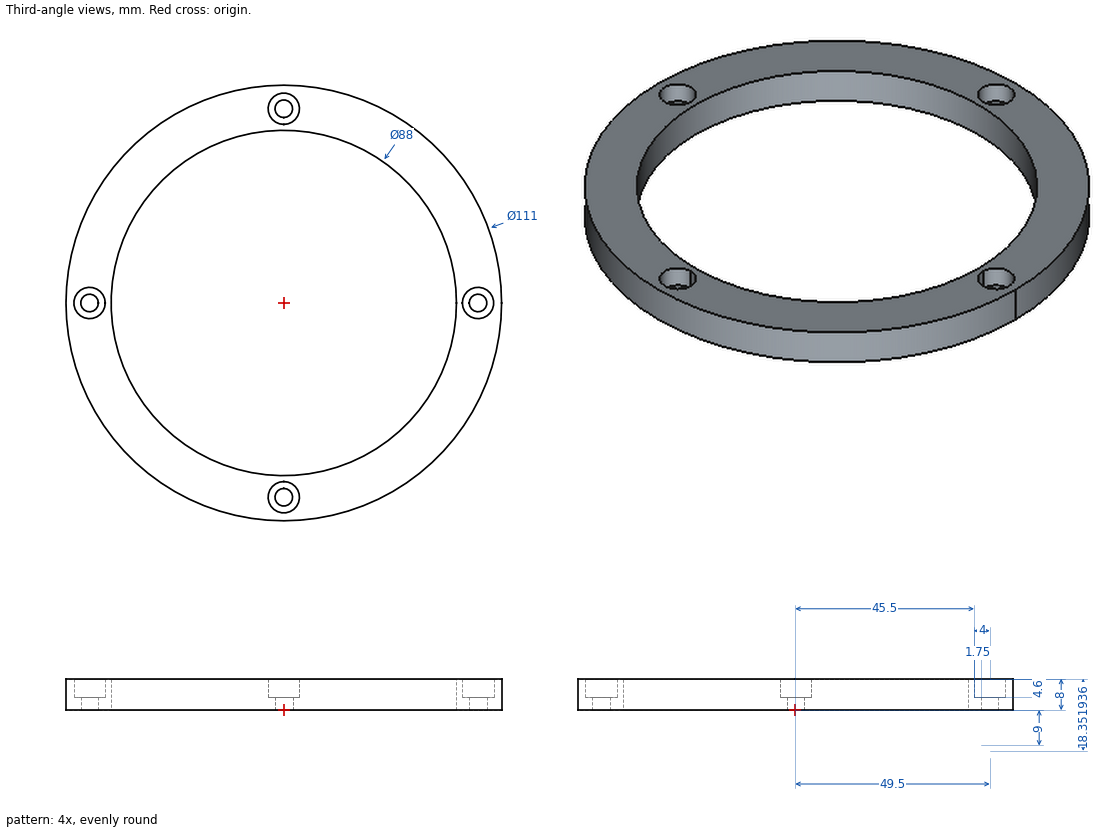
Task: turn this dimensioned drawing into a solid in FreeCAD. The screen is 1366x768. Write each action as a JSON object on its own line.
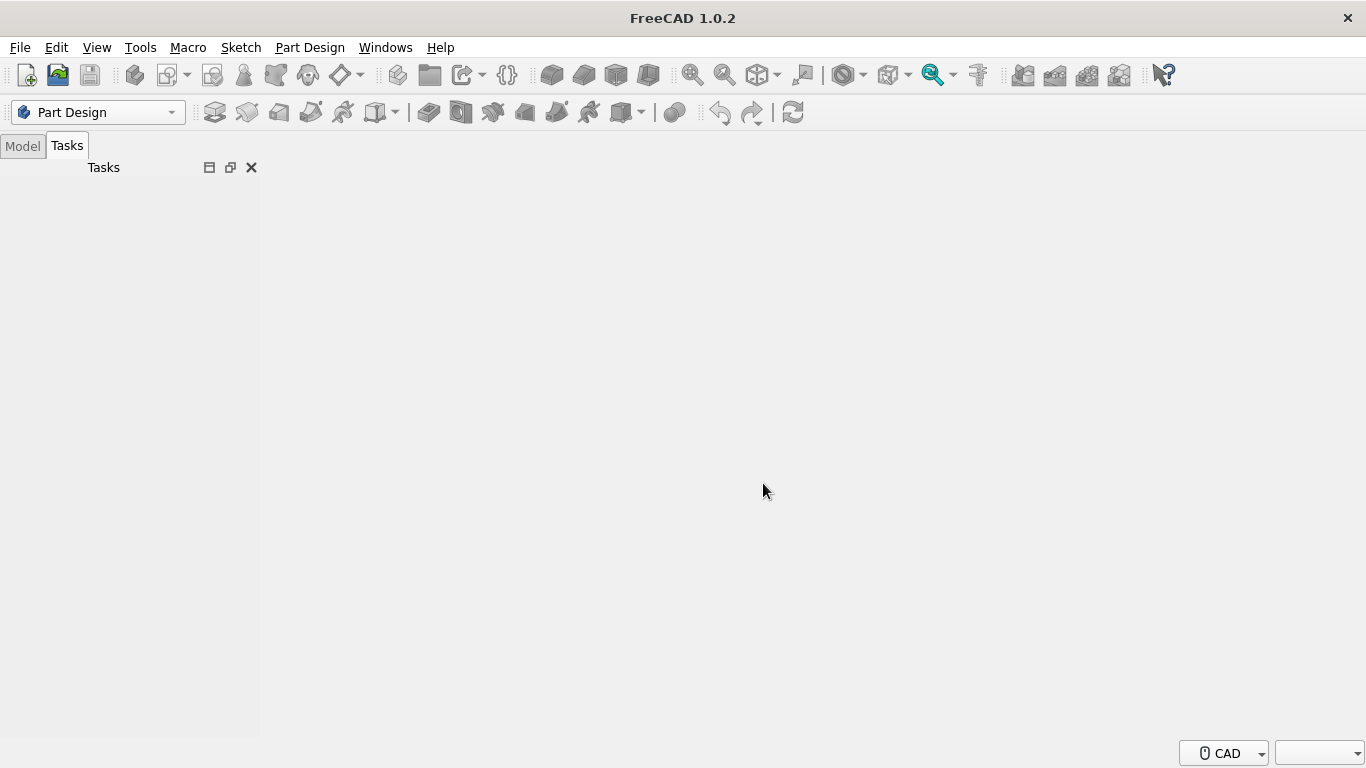
{"action": "left_click", "coordinate": [26, 76]}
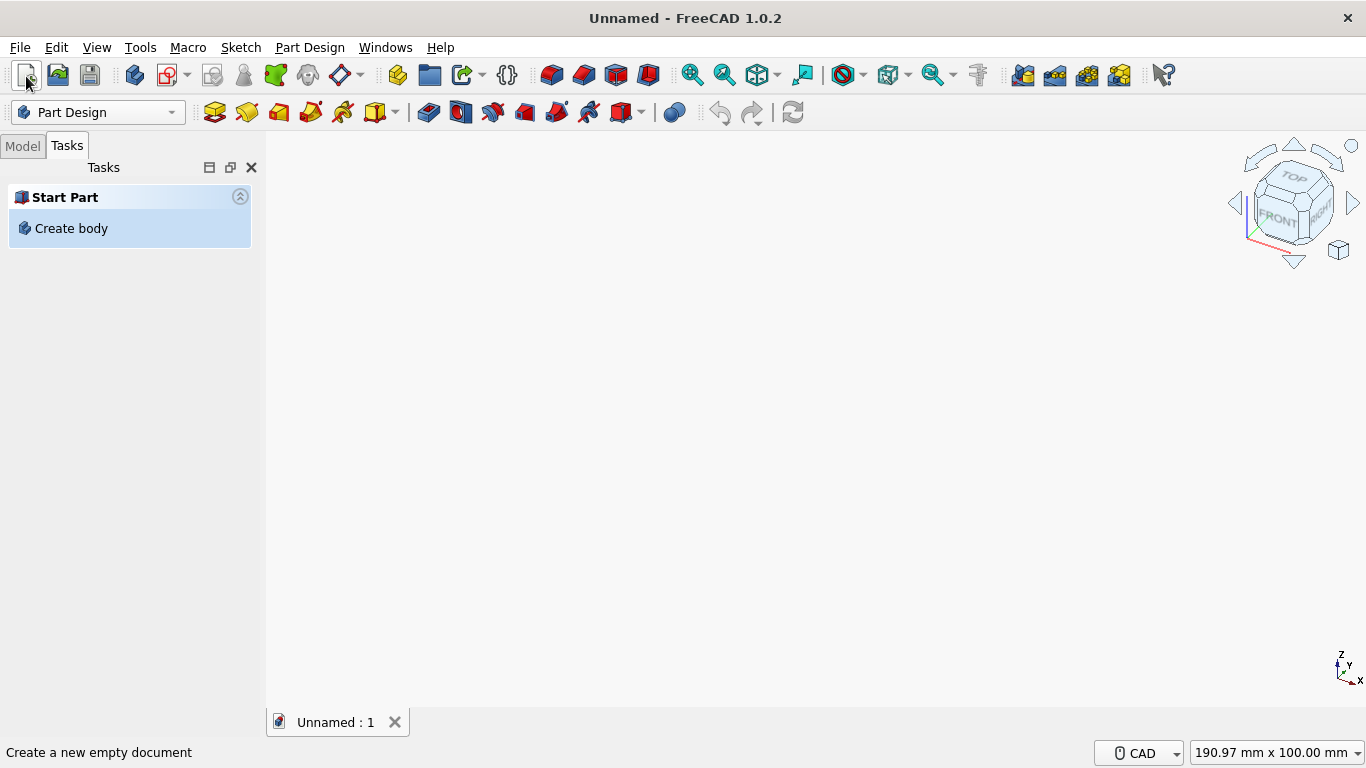
{"action": "left_click", "coordinate": [168, 76]}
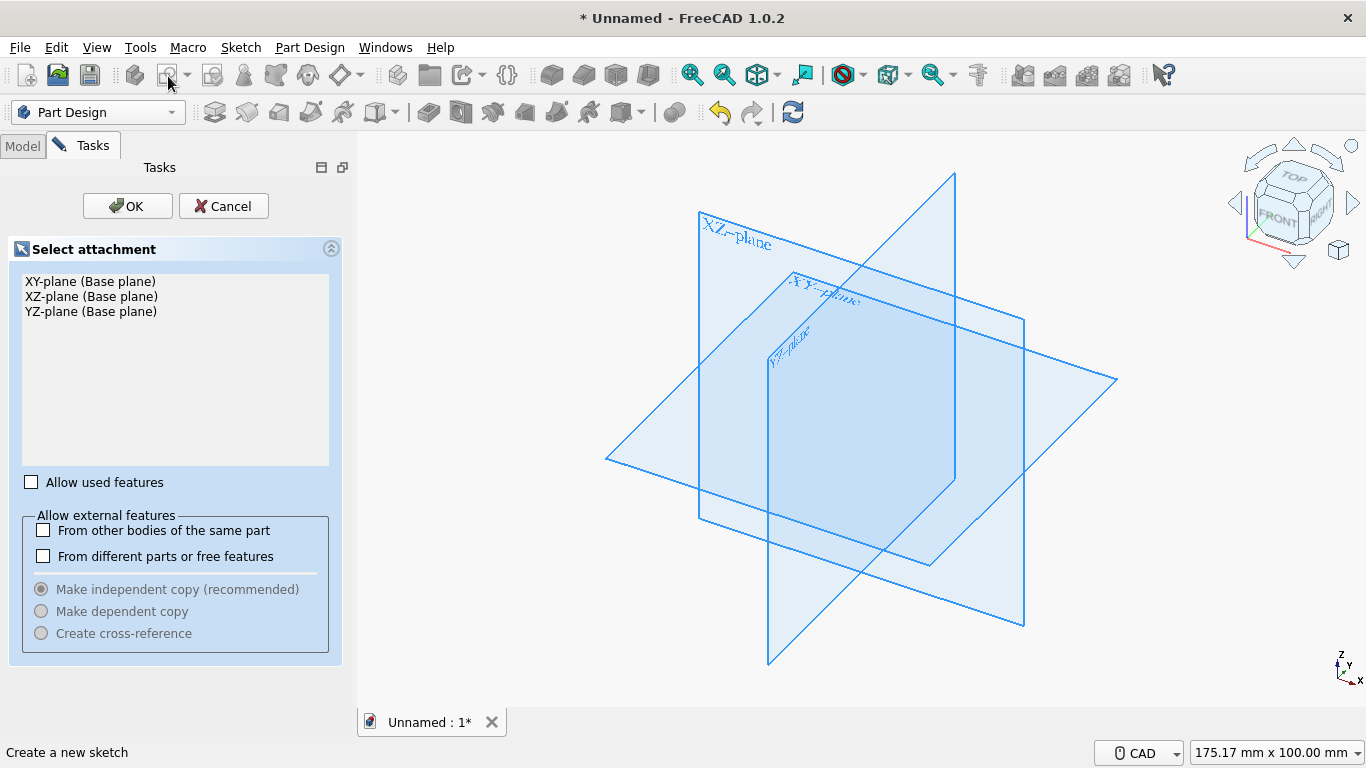
{"action": "left_click", "coordinate": [82, 282]}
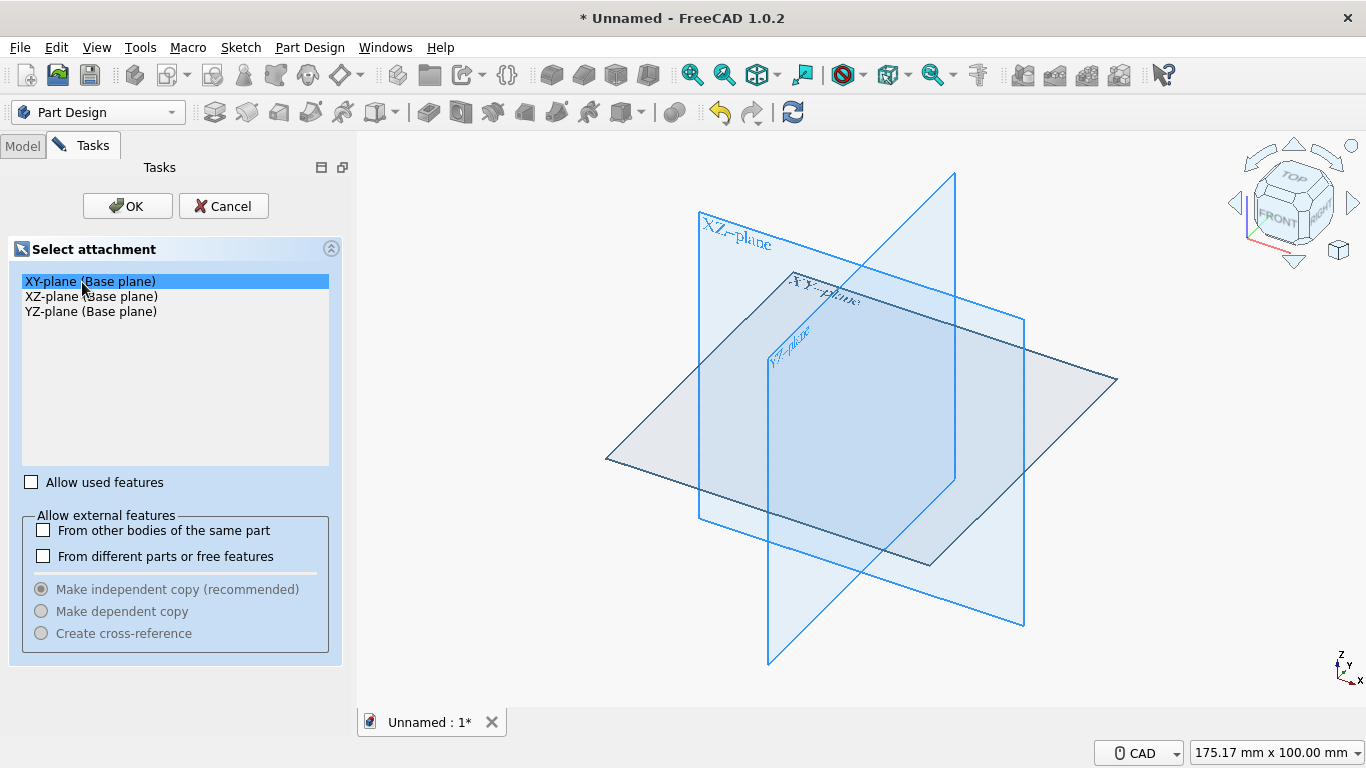
{"action": "left_click", "coordinate": [128, 206]}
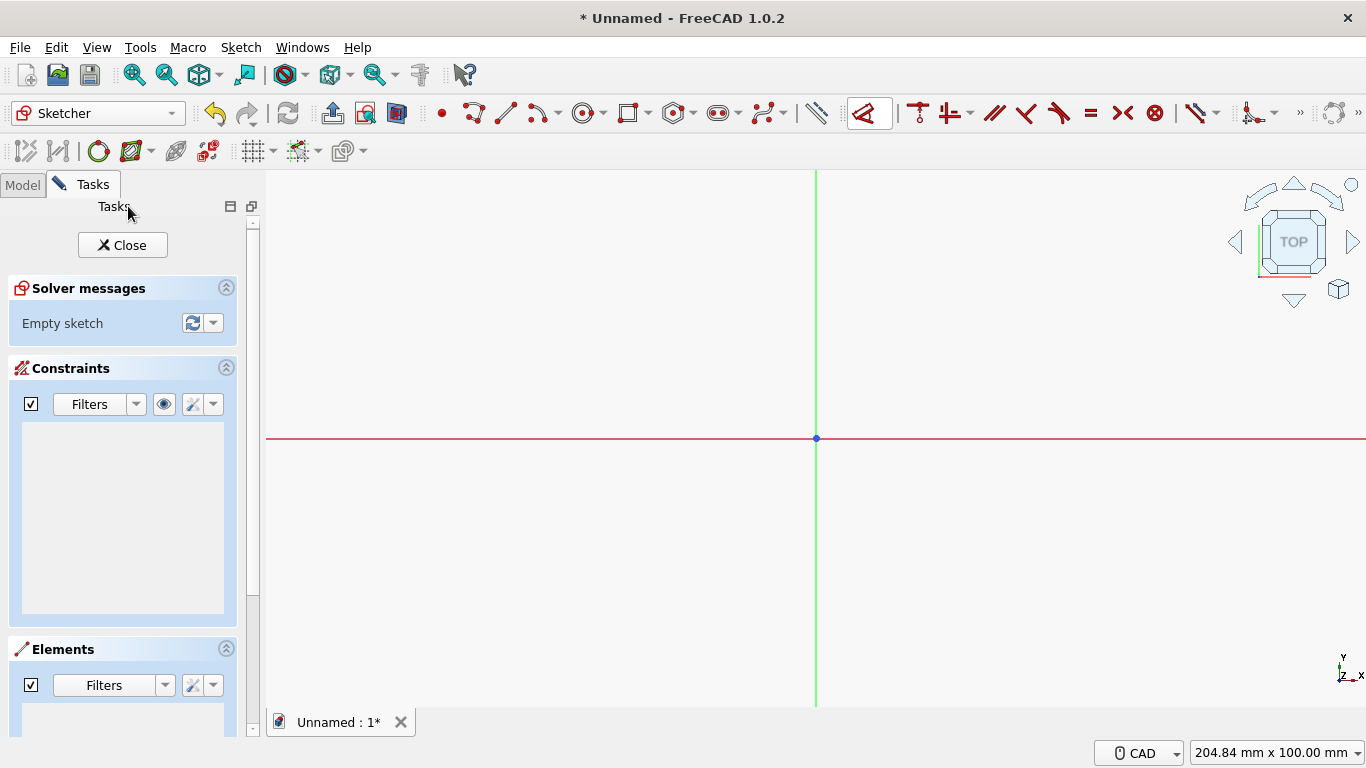
{"action": "scroll", "coordinate": [664, 438], "scroll_direction": "down", "scroll_amount": 3}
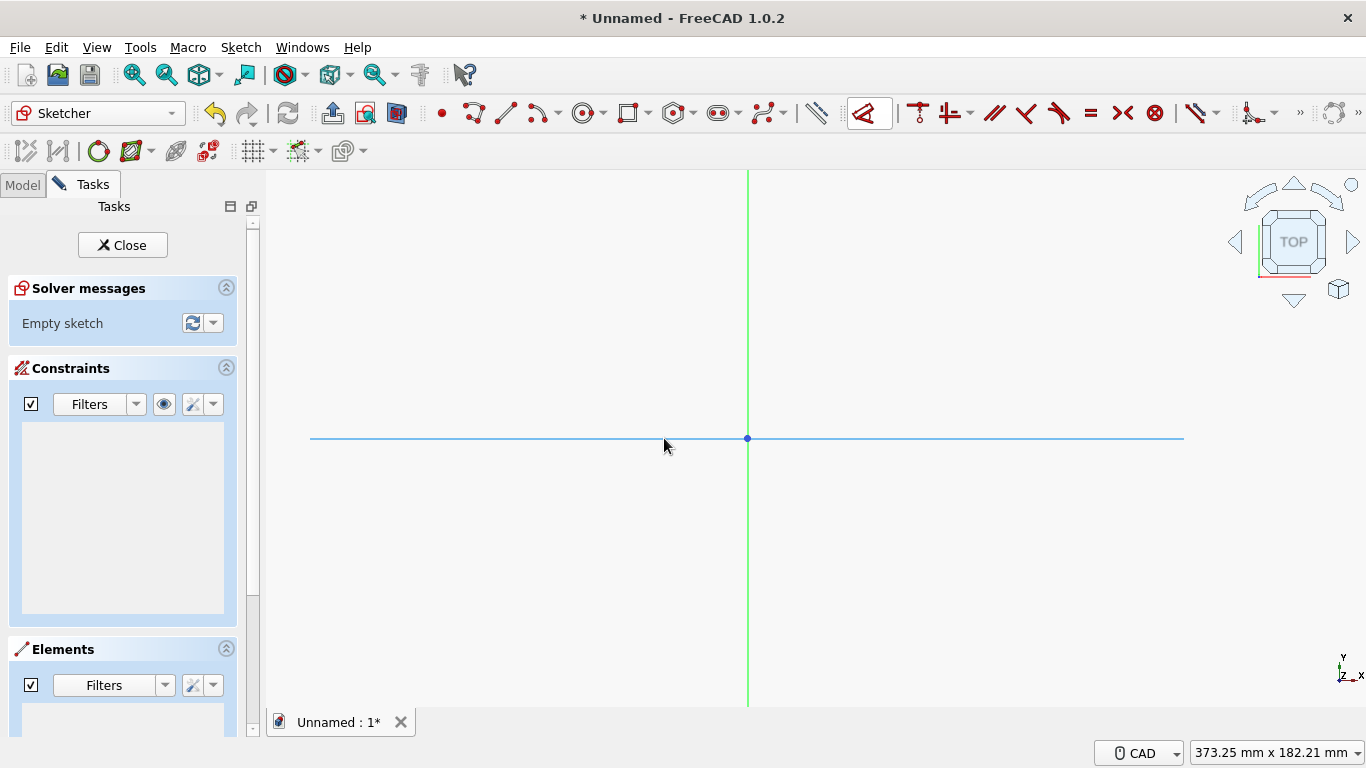
{"action": "key", "text": "g c"}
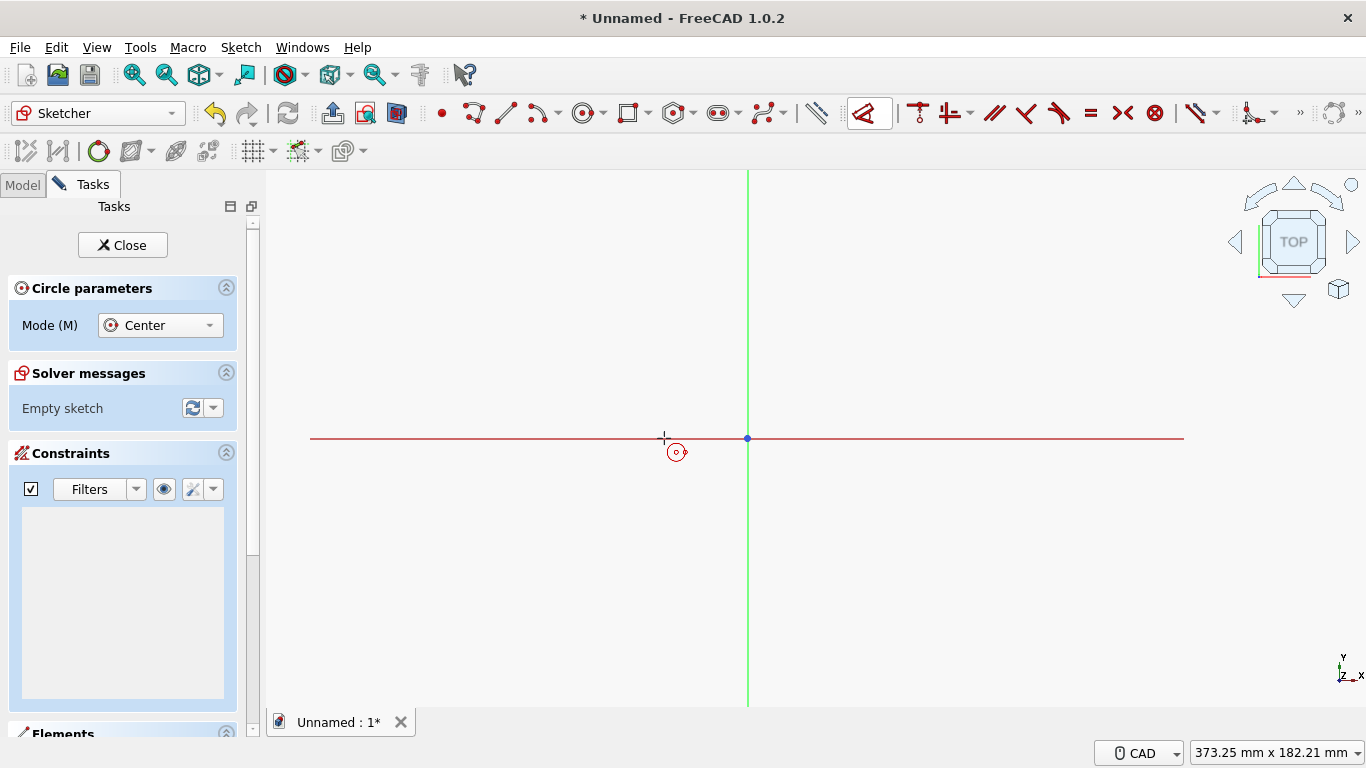
{"action": "left_click", "coordinate": [748, 438]}
{"action": "mouse_move", "coordinate": [863, 323]}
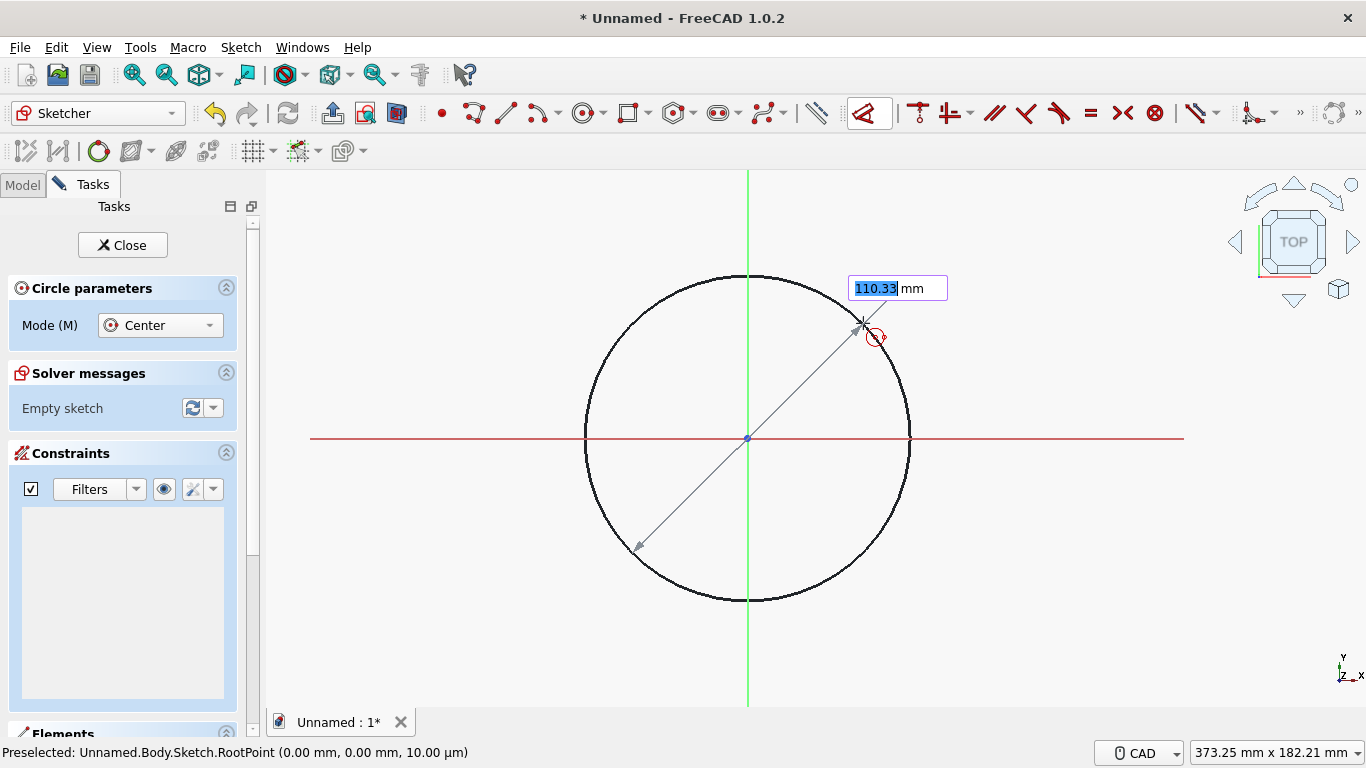
{"action": "type", "text": "111"}
{"action": "key", "text": "Return"}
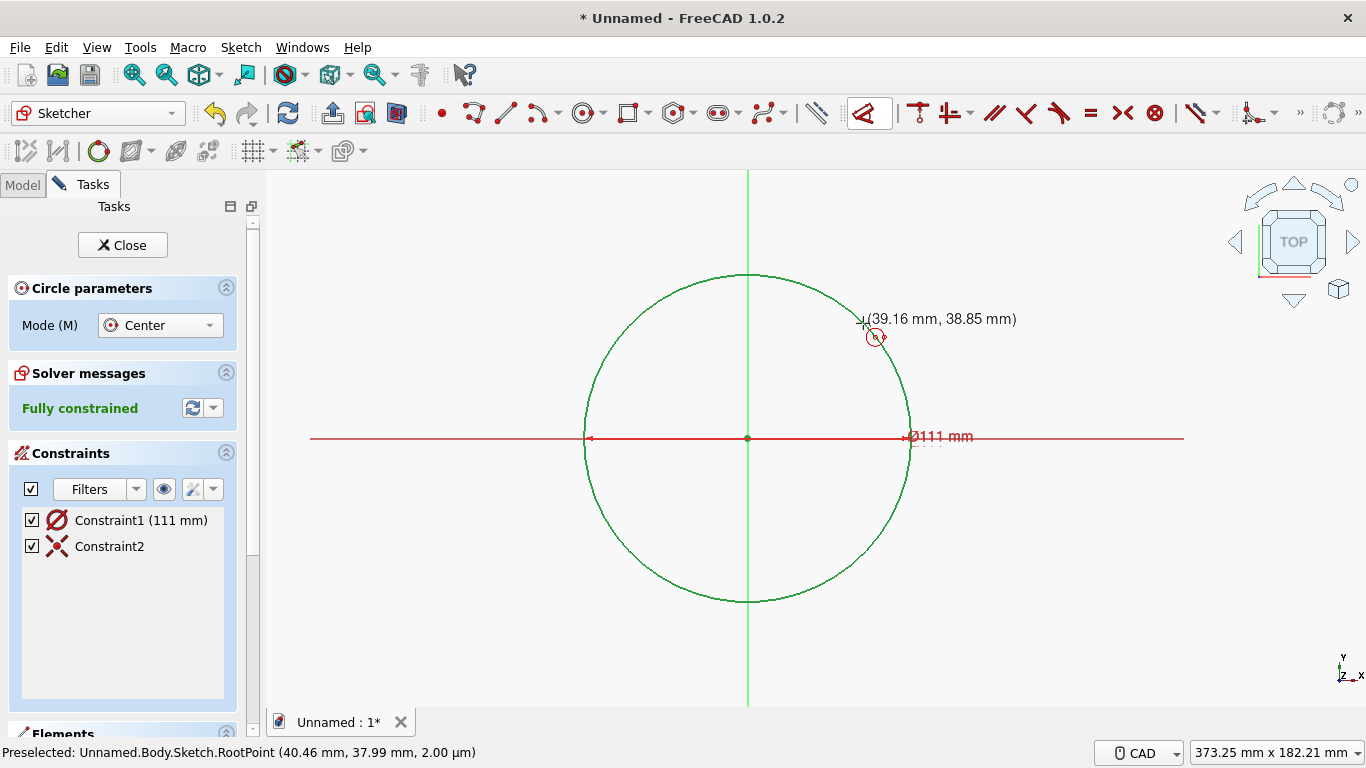
{"action": "left_click", "coordinate": [748, 438]}
{"action": "mouse_move", "coordinate": [839, 347]}